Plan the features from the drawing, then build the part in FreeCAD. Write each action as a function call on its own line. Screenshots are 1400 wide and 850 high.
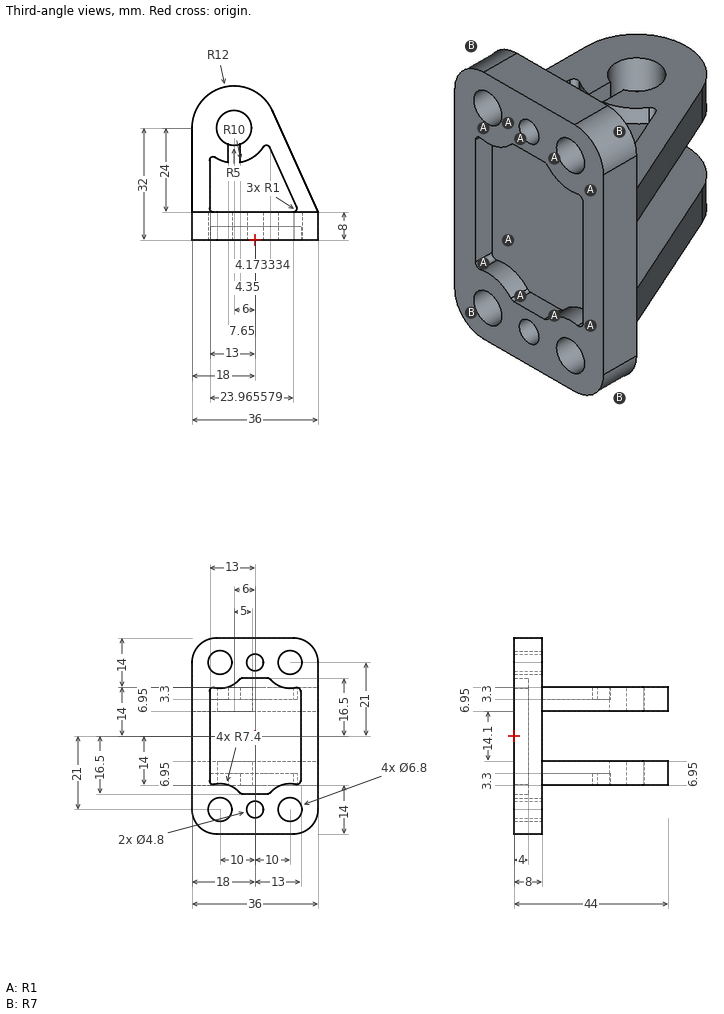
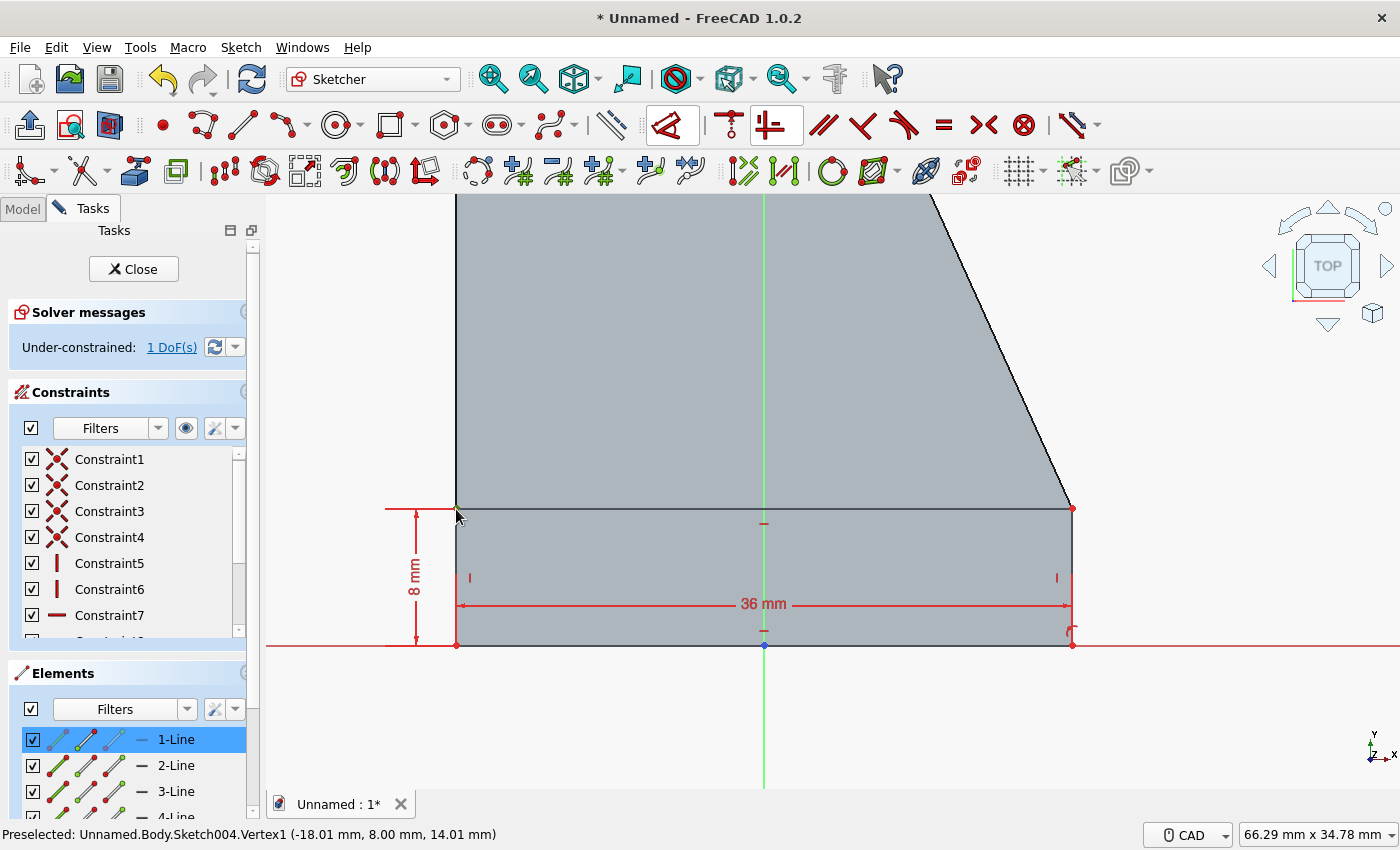
key(l)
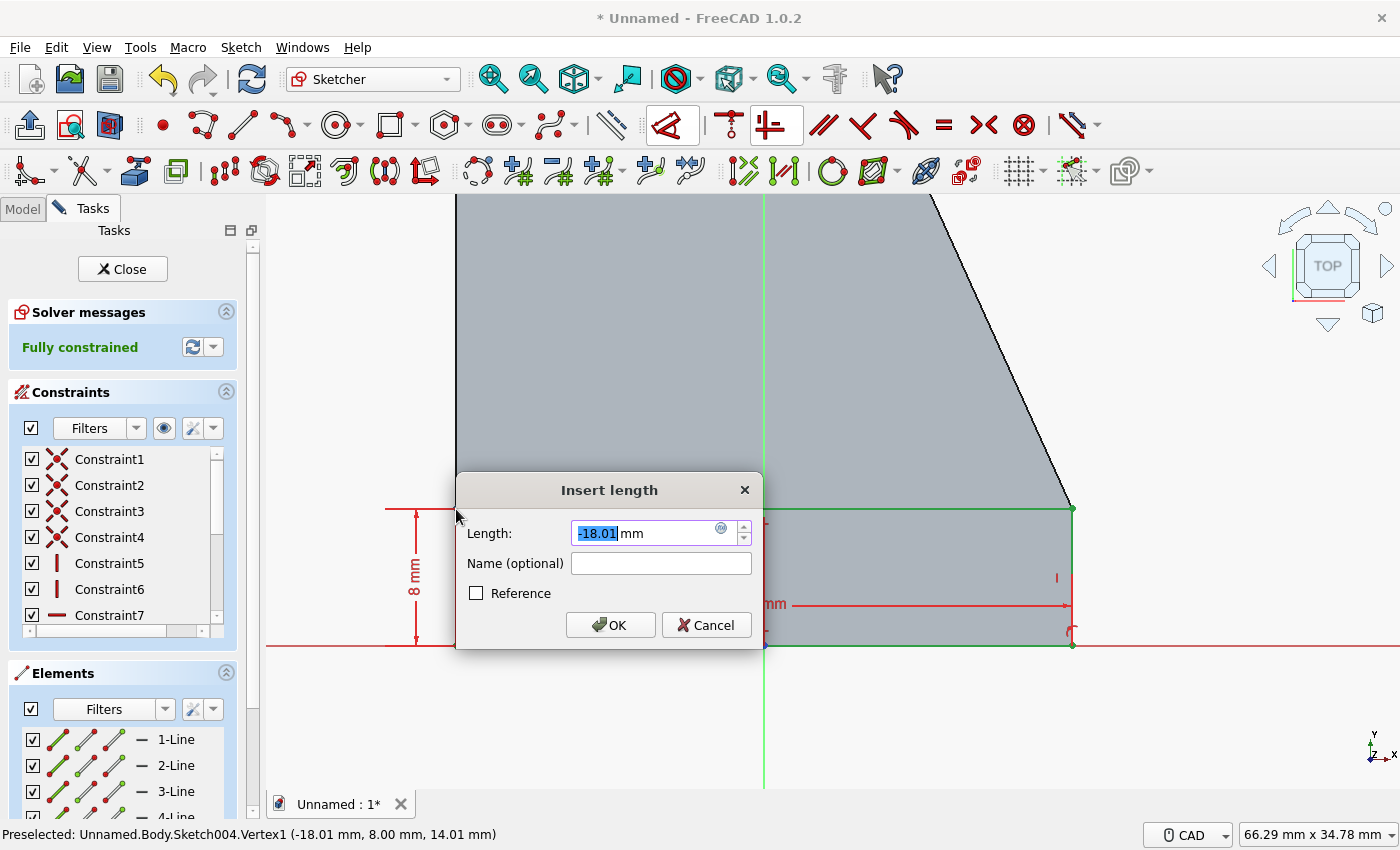
text(-18)
key(Return)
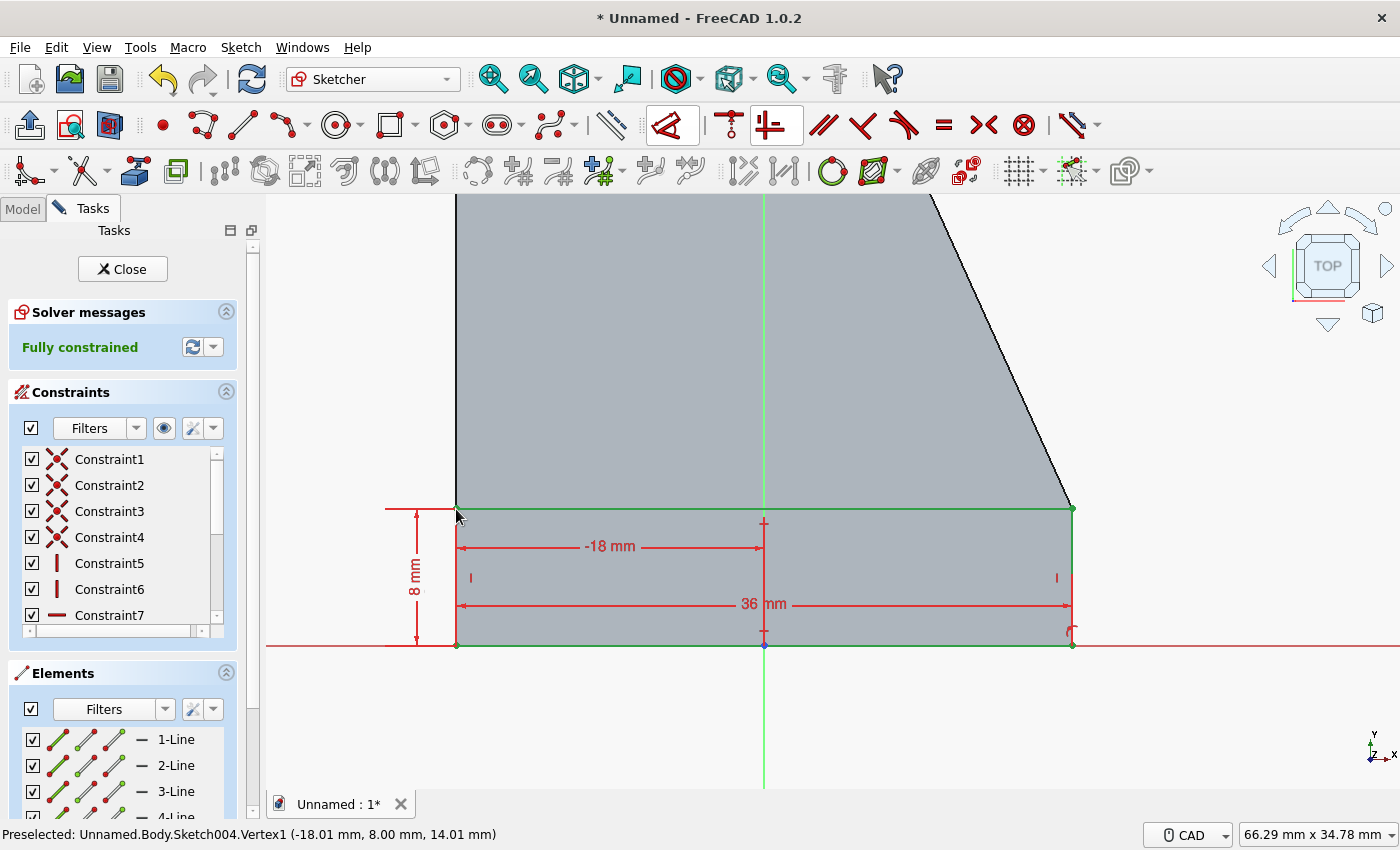
click(123, 269)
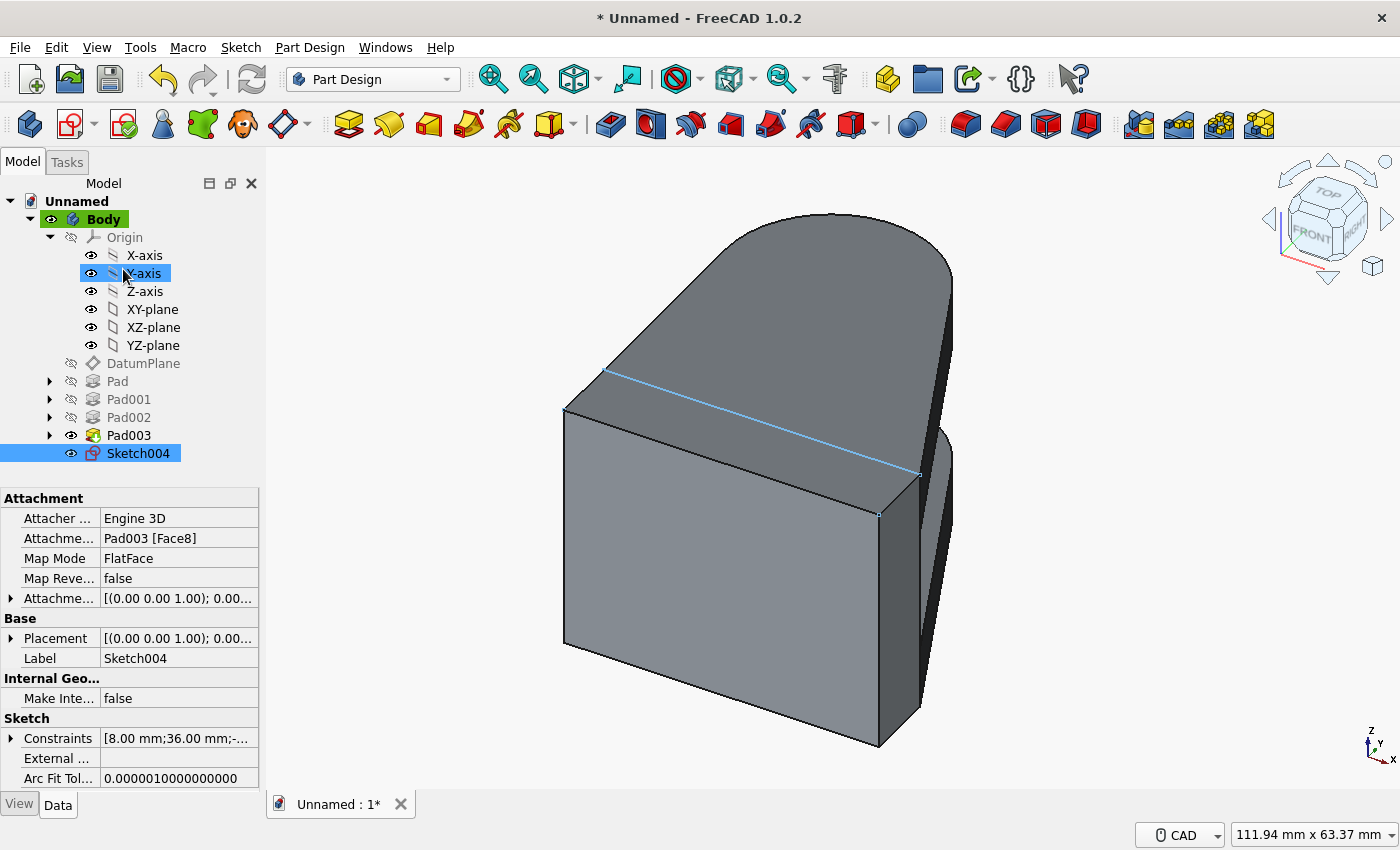
click(350, 124)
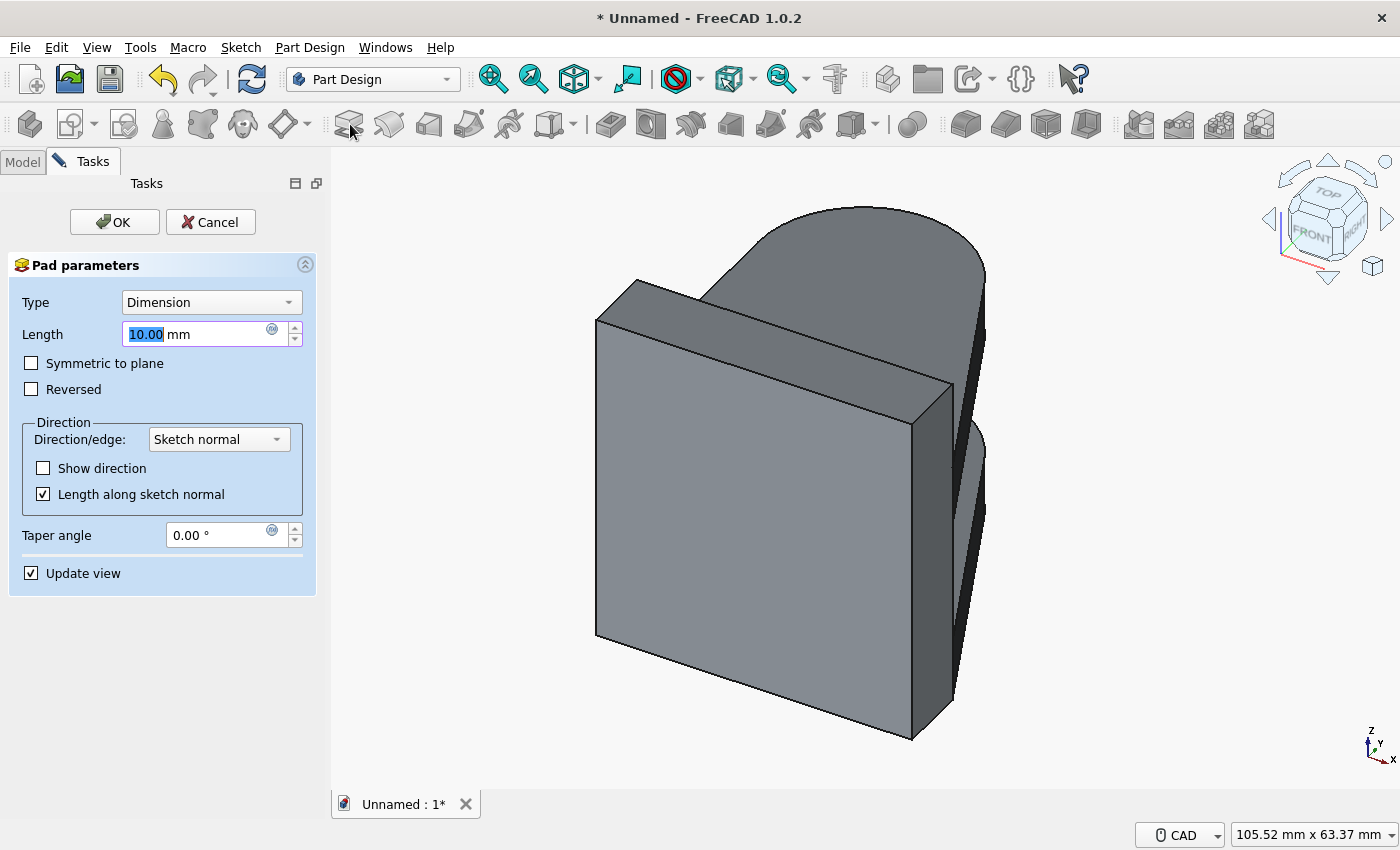
text(14)
key(Tab)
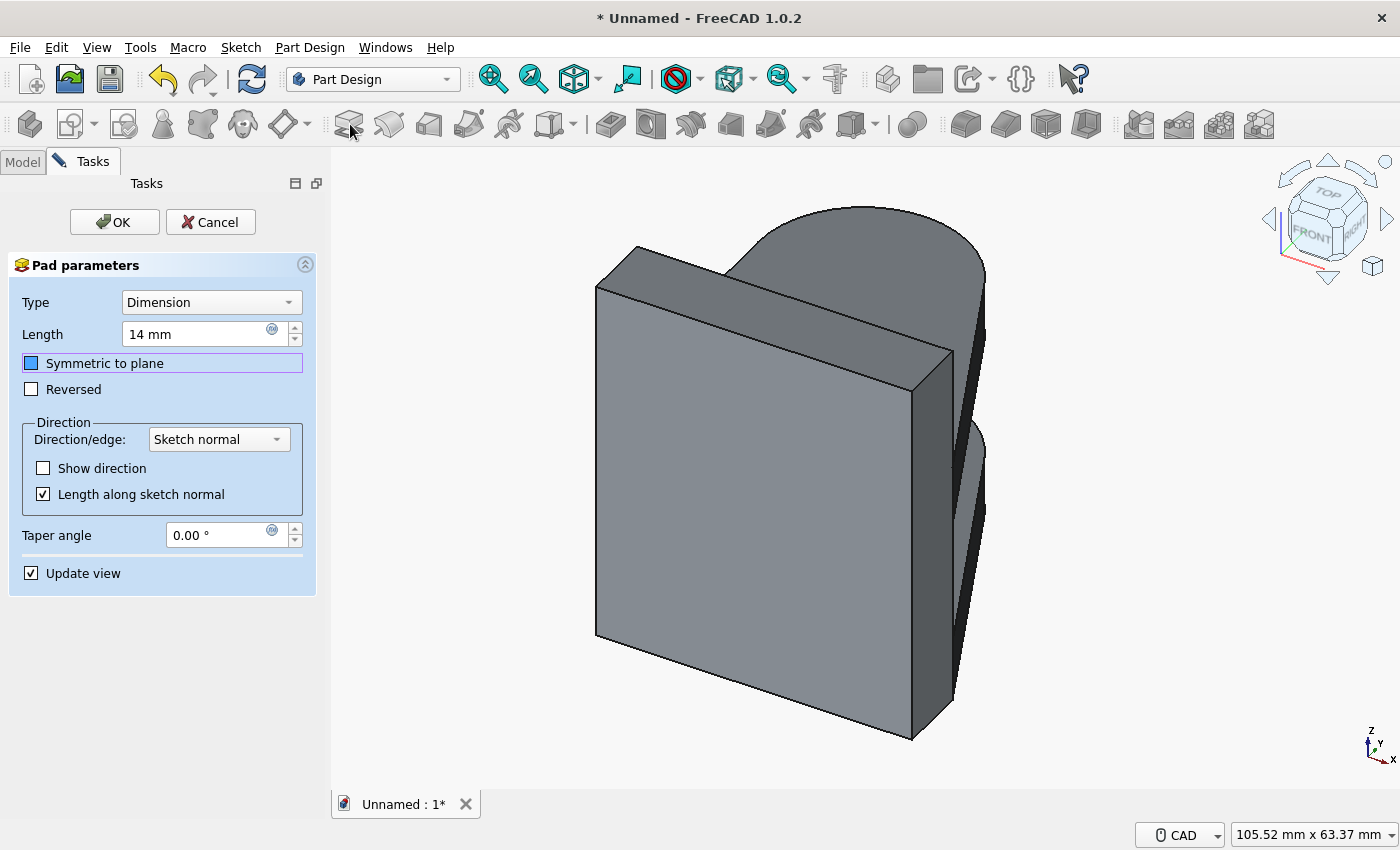
click(115, 222)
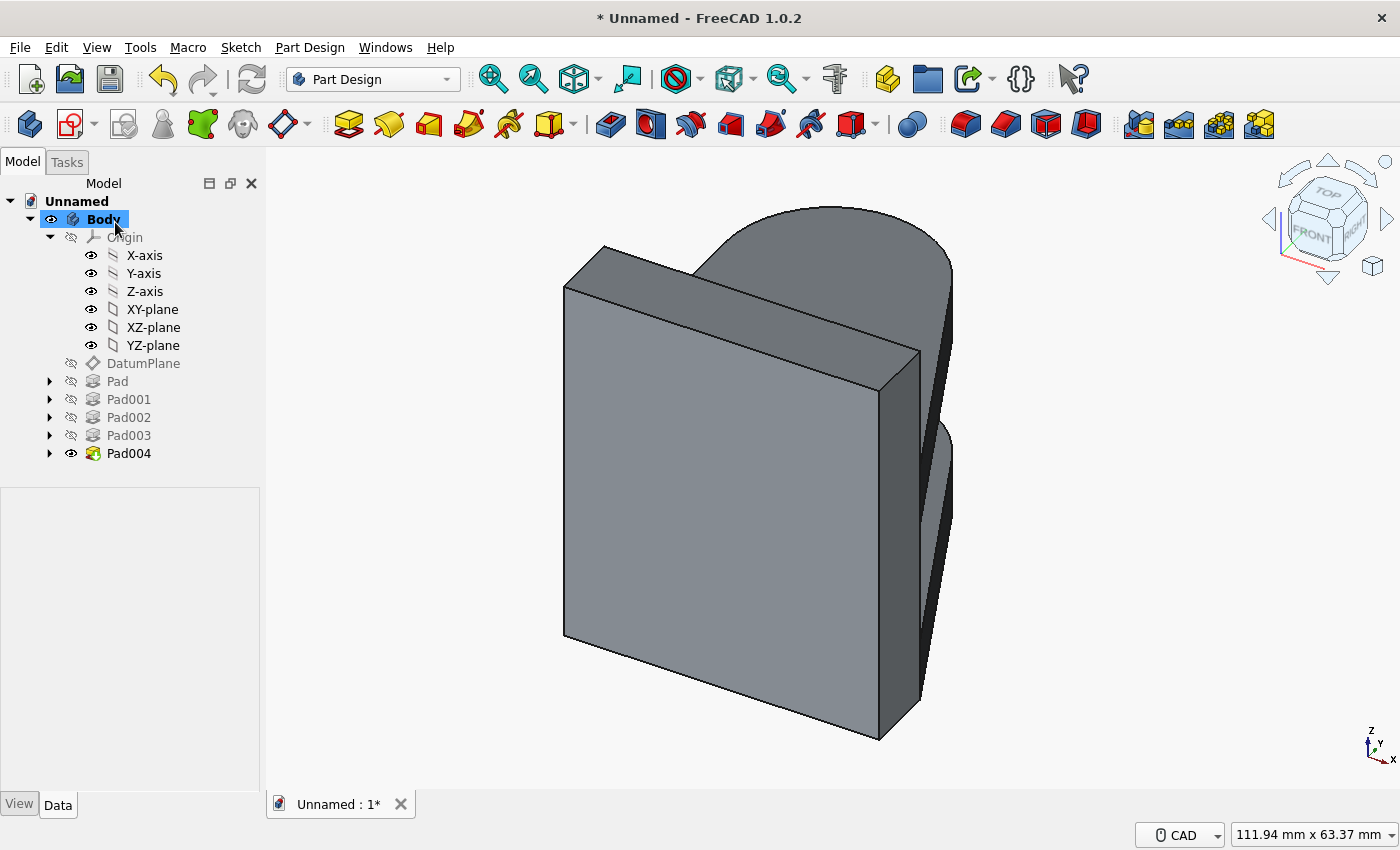
key(v)
key(f)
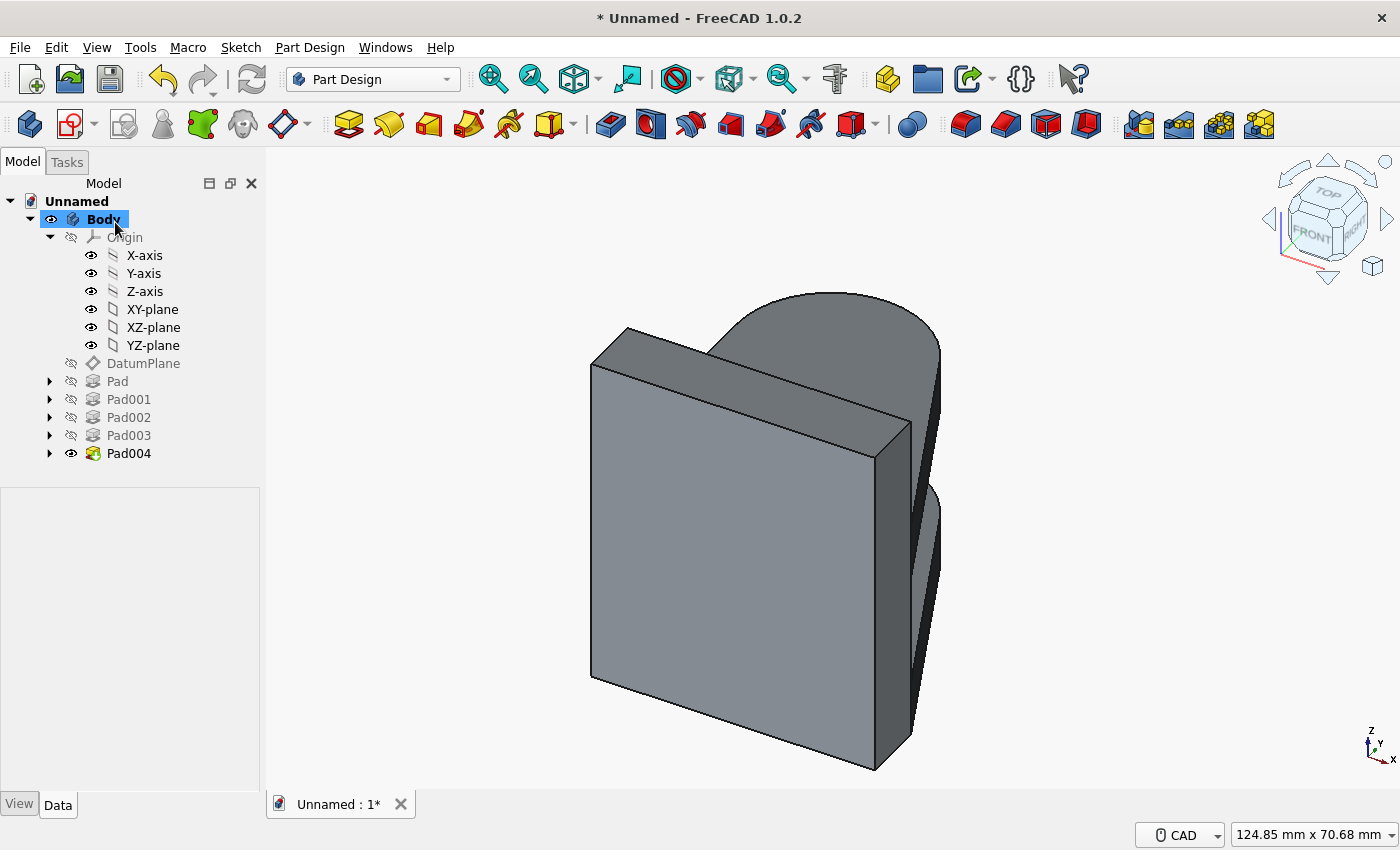
click(834, 360)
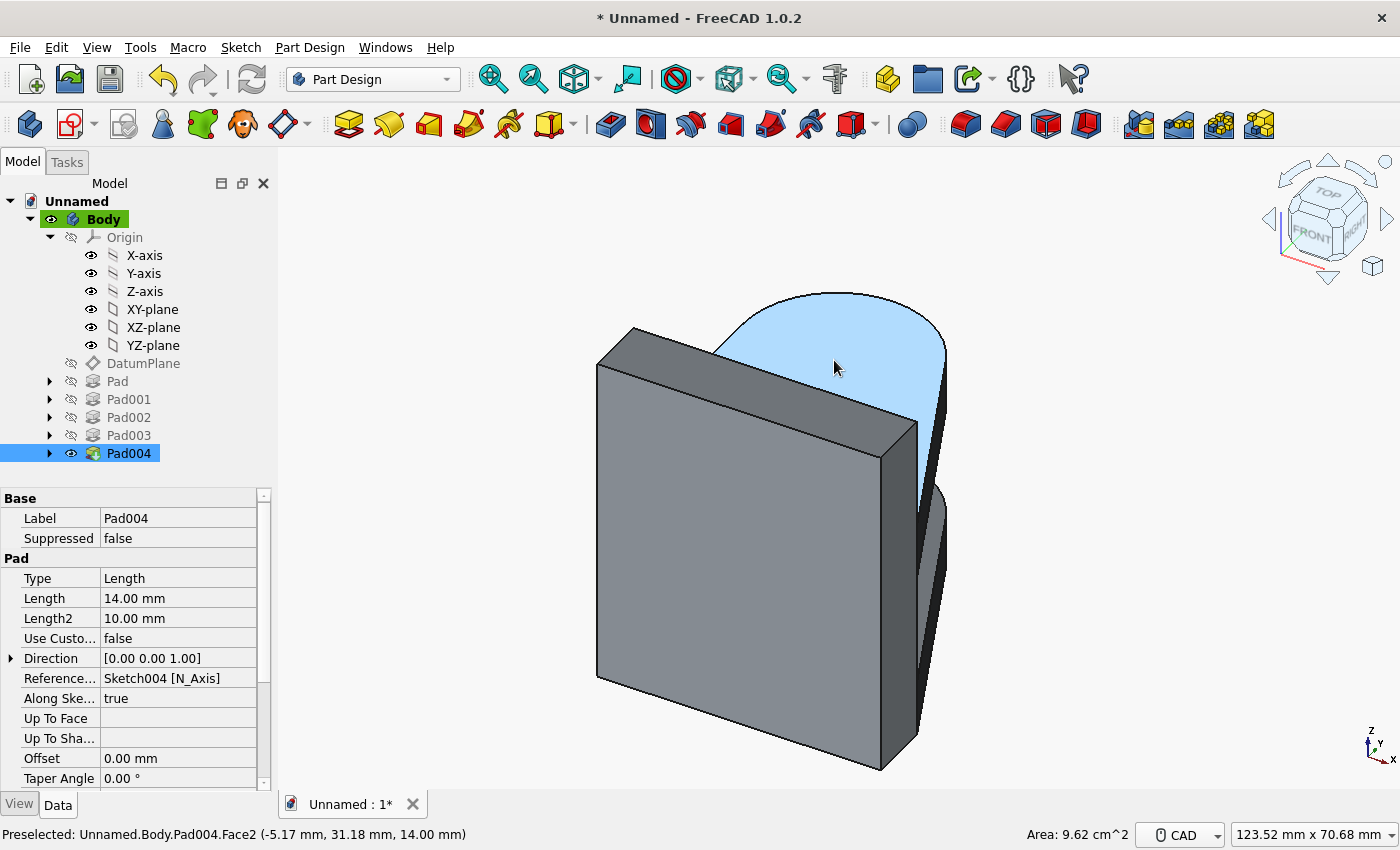
click(70, 124)